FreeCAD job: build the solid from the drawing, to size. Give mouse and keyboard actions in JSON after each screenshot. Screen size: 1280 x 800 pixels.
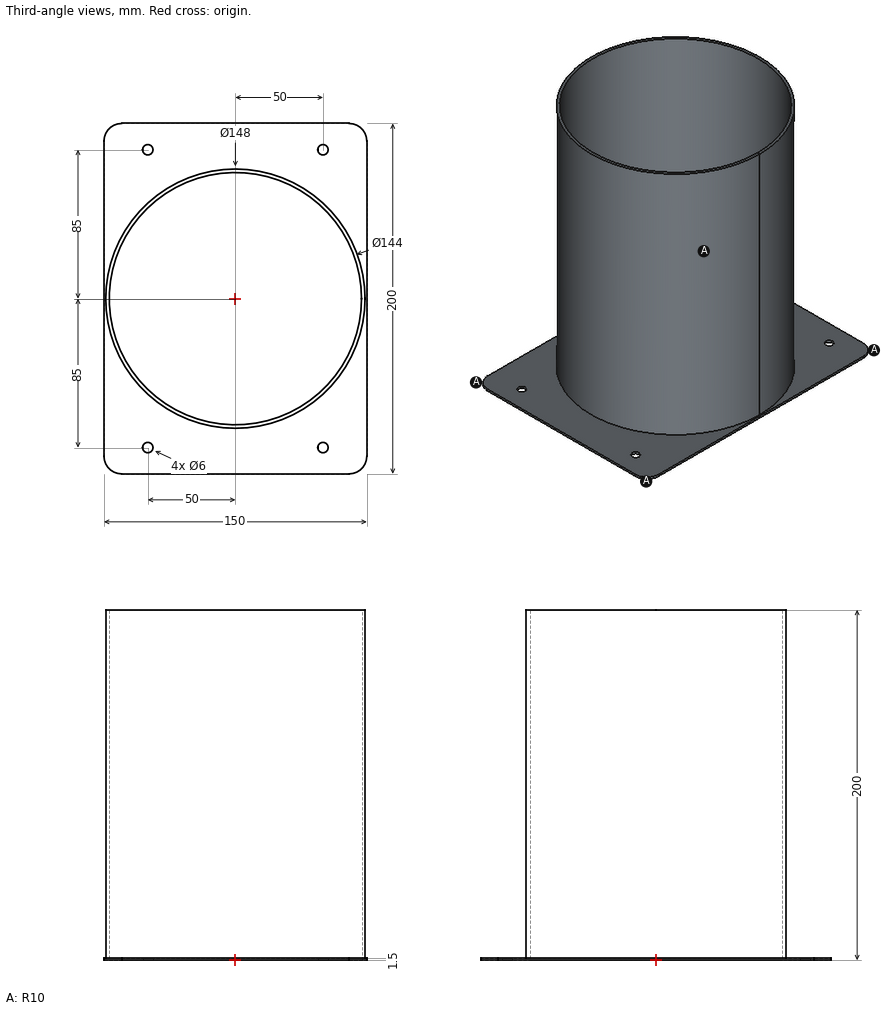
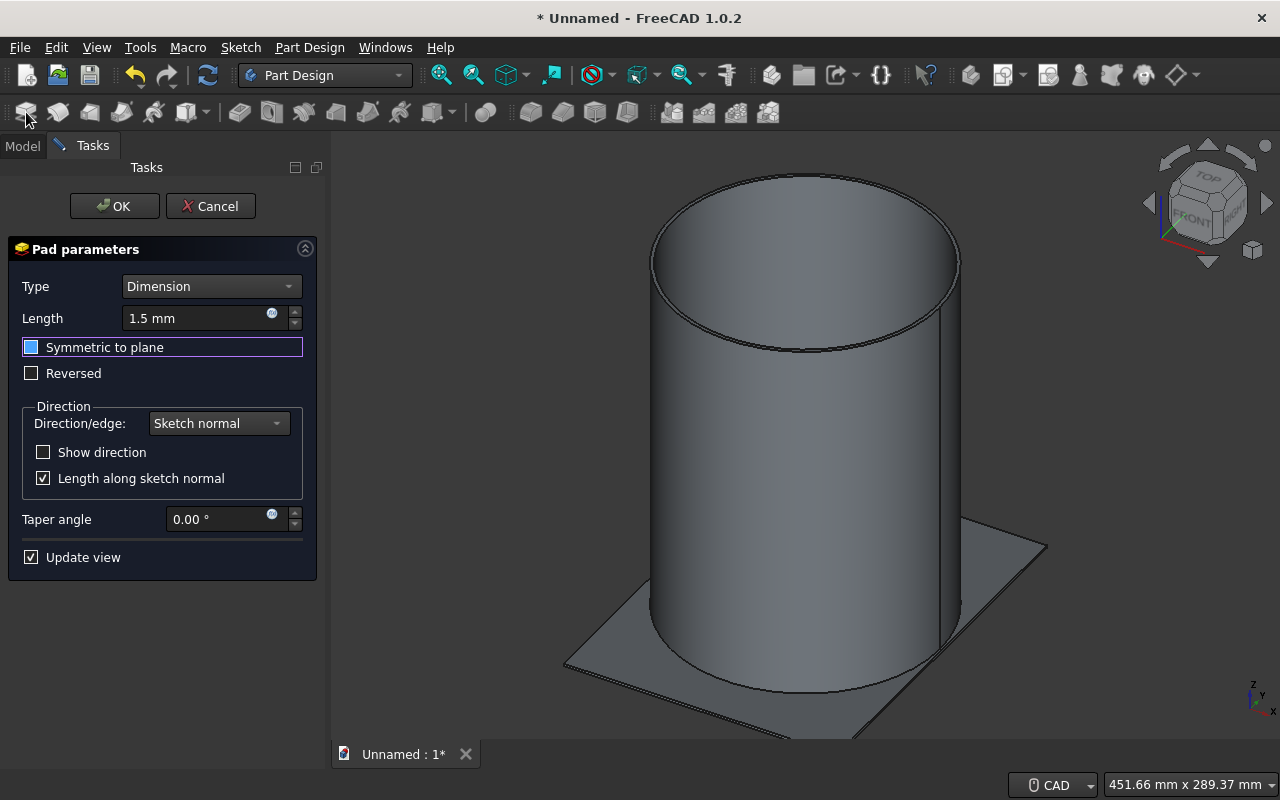
{"action": "left_click", "coordinate": [115, 206]}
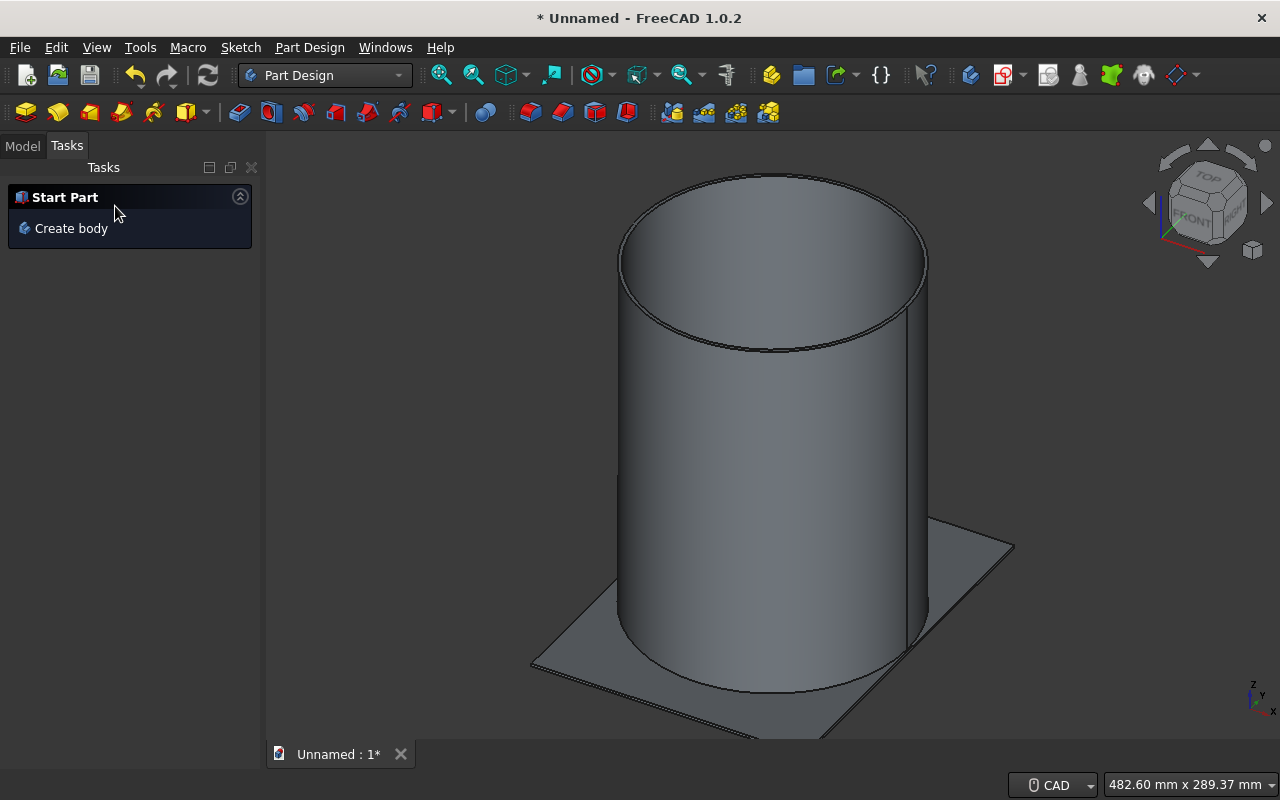
{"action": "left_click", "coordinate": [442, 76]}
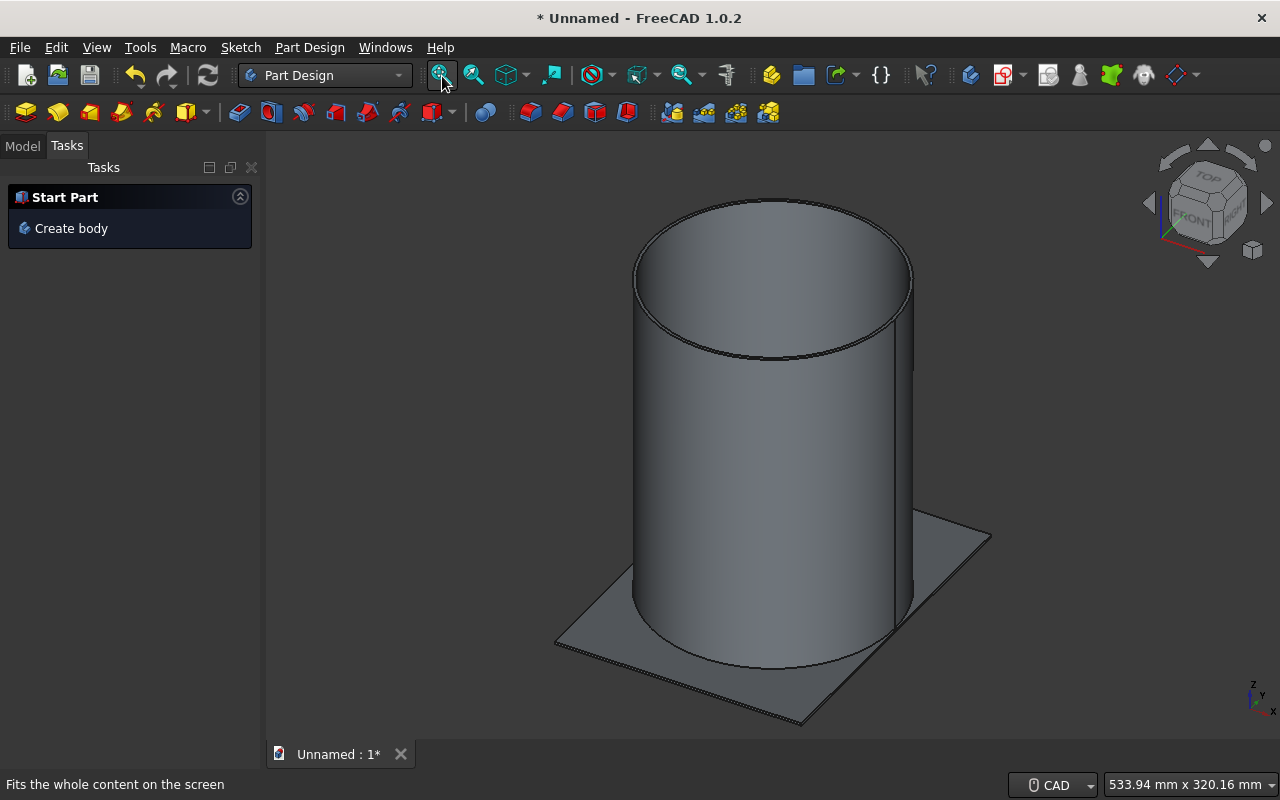
{"action": "scroll", "coordinate": [745, 453], "scroll_direction": "up", "scroll_amount": 14}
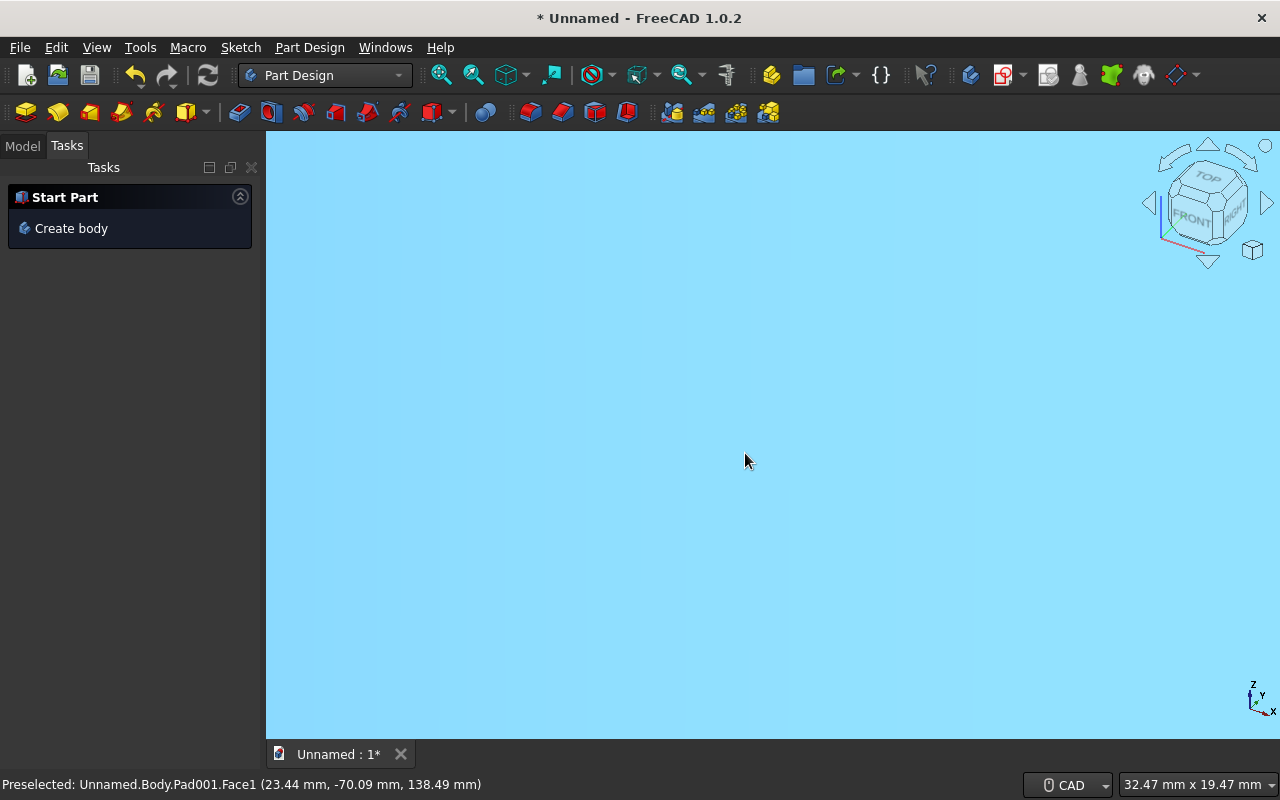
{"action": "left_click", "coordinate": [442, 76]}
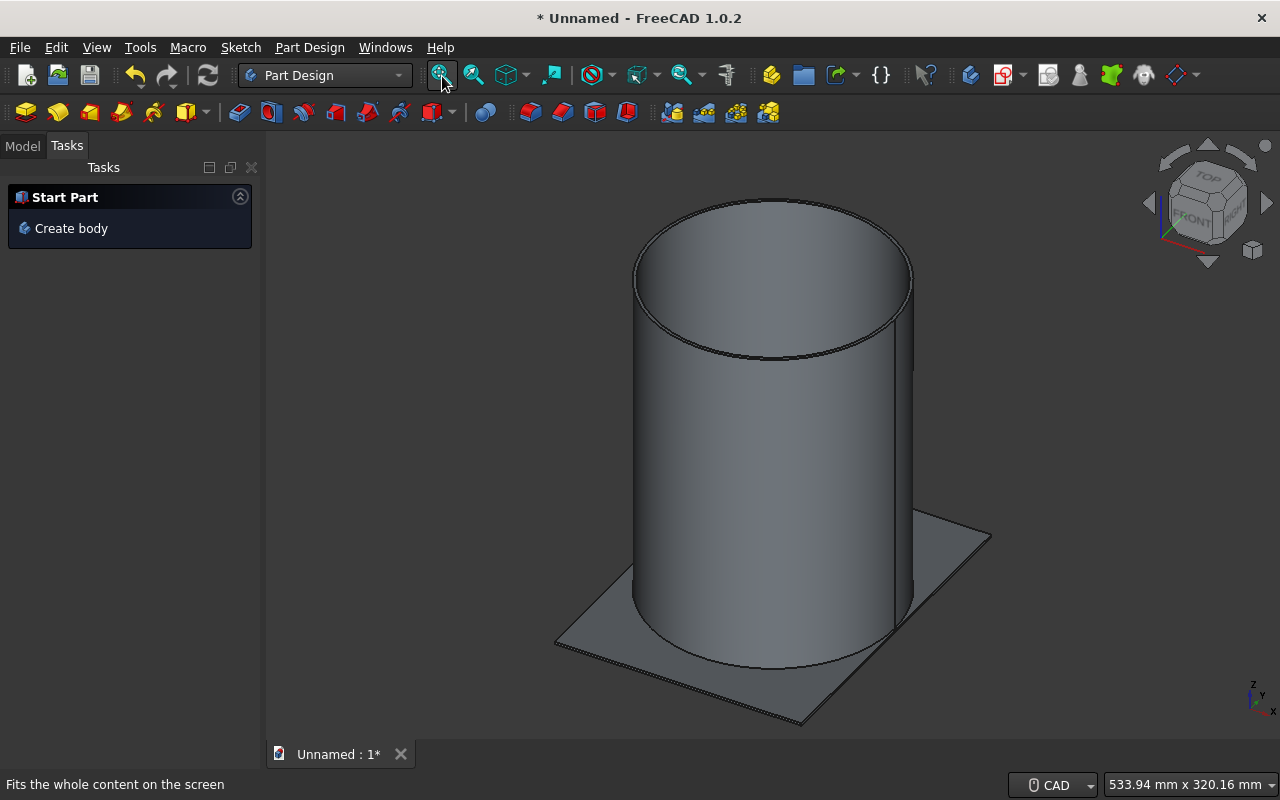
{"action": "key", "text": "0"}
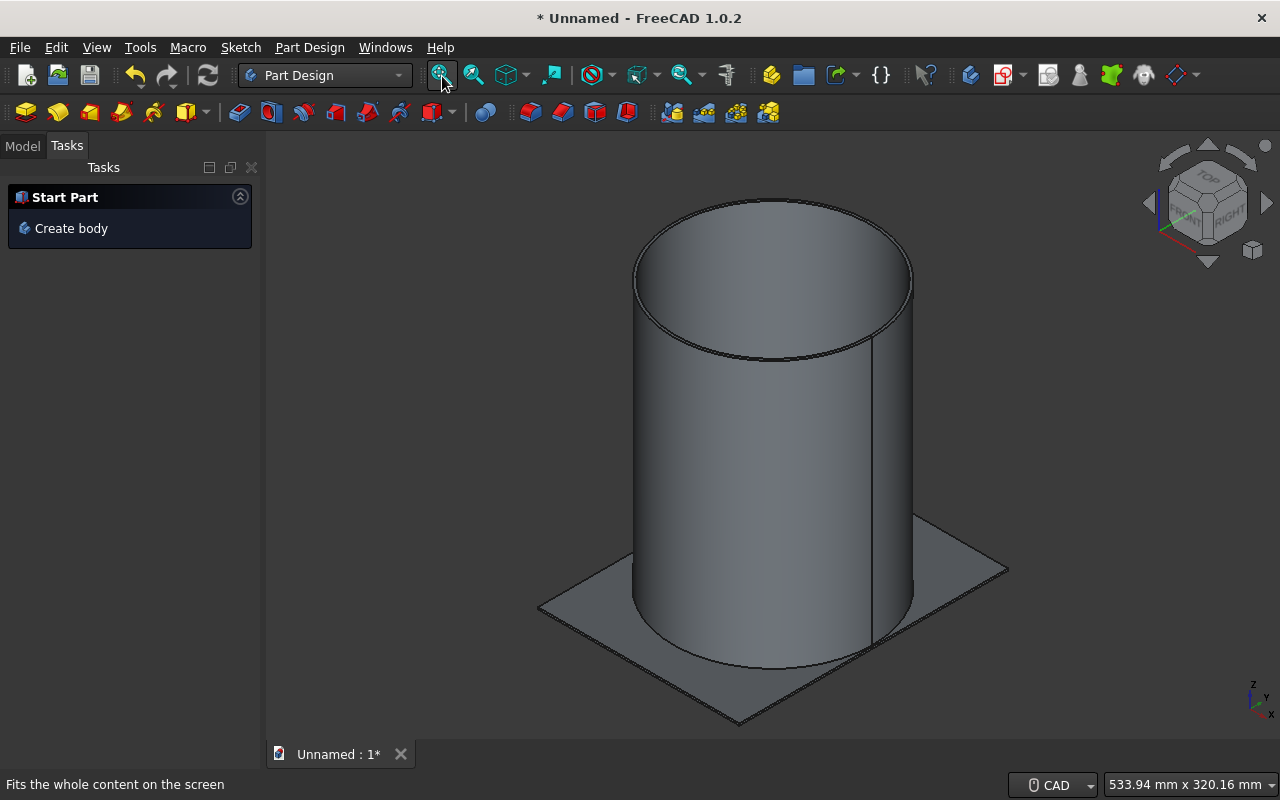
{"action": "scroll", "coordinate": [807, 452], "scroll_direction": "up", "scroll_amount": 14}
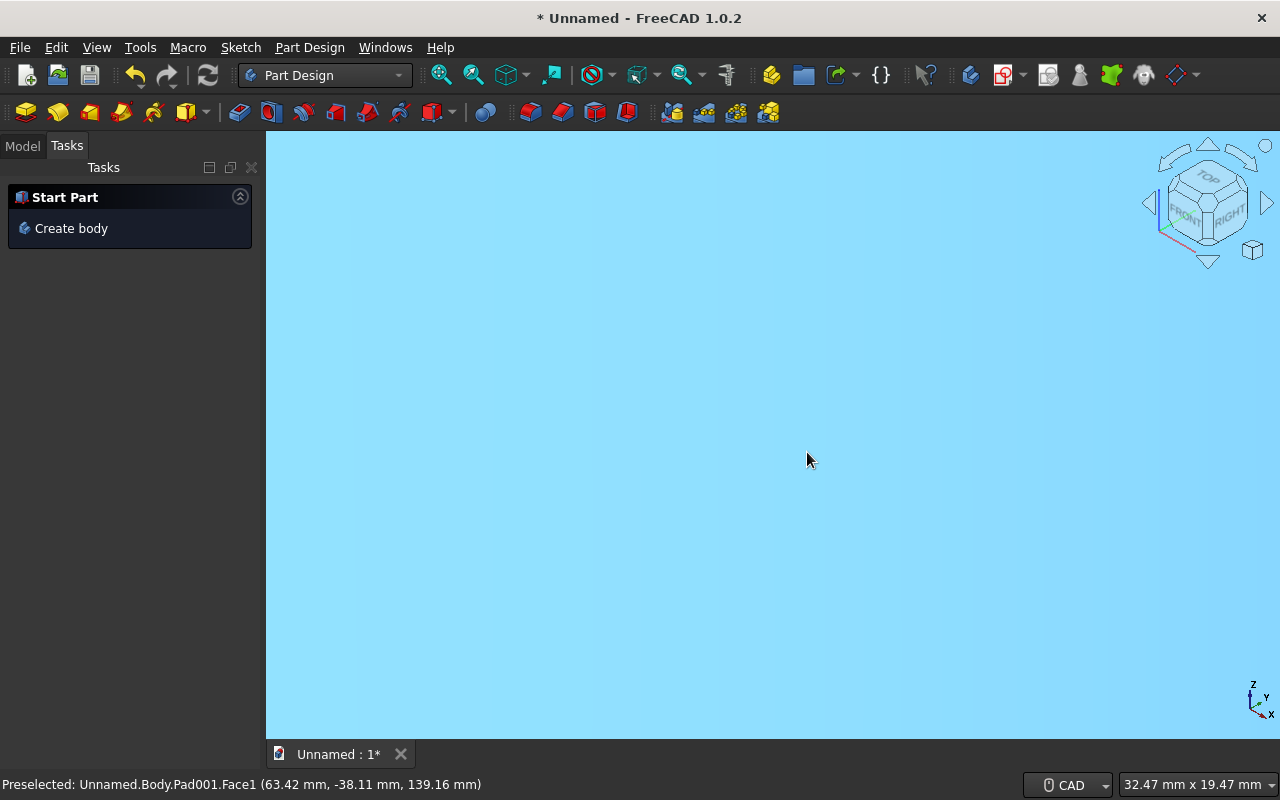
{"action": "left_click", "coordinate": [442, 76]}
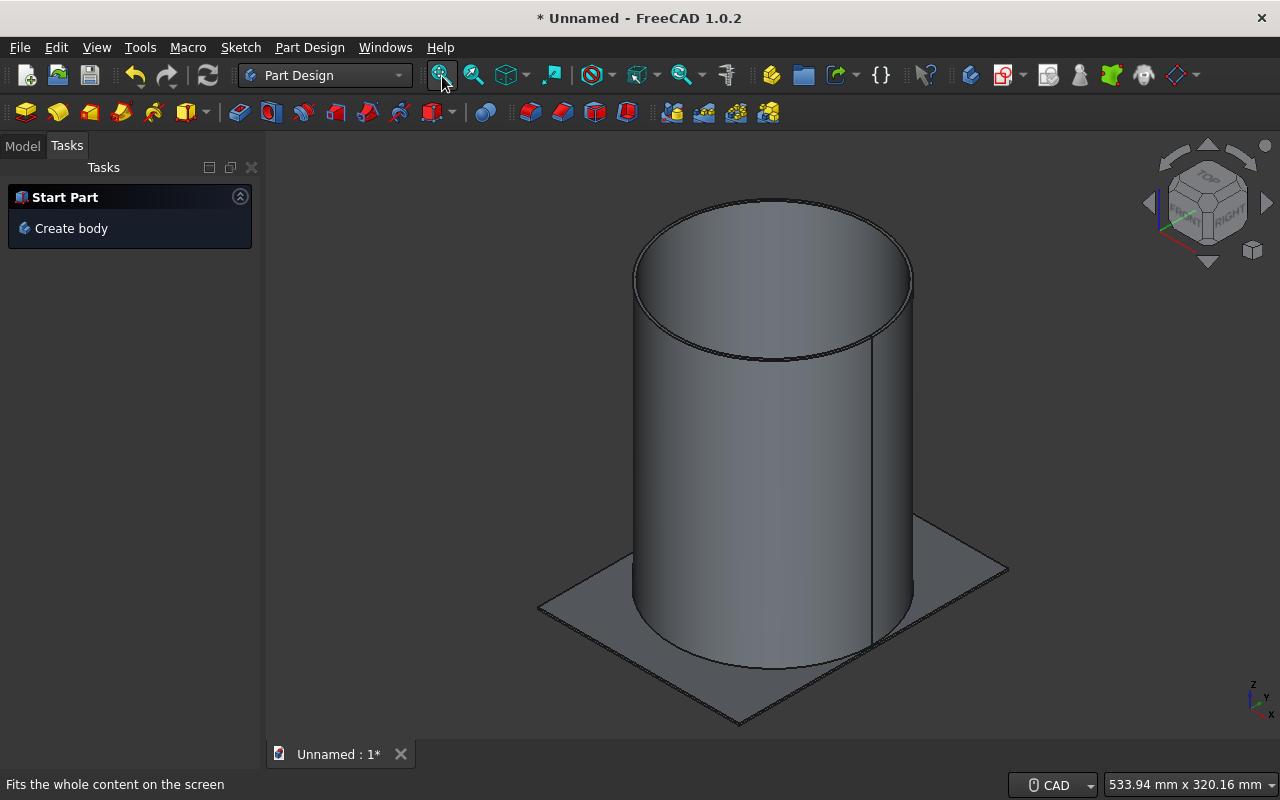
{"action": "key", "text": "2"}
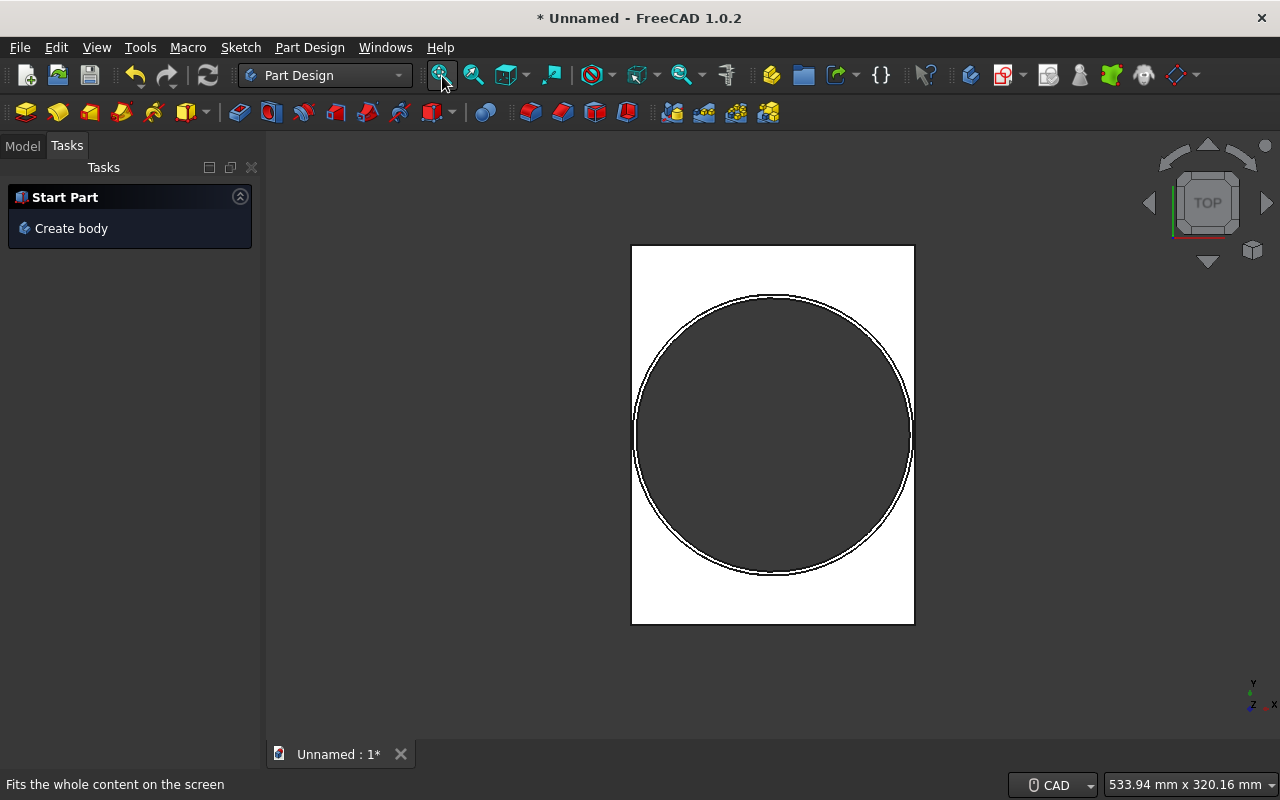
{"action": "scroll", "coordinate": [631, 244], "scroll_direction": "up", "scroll_amount": 14}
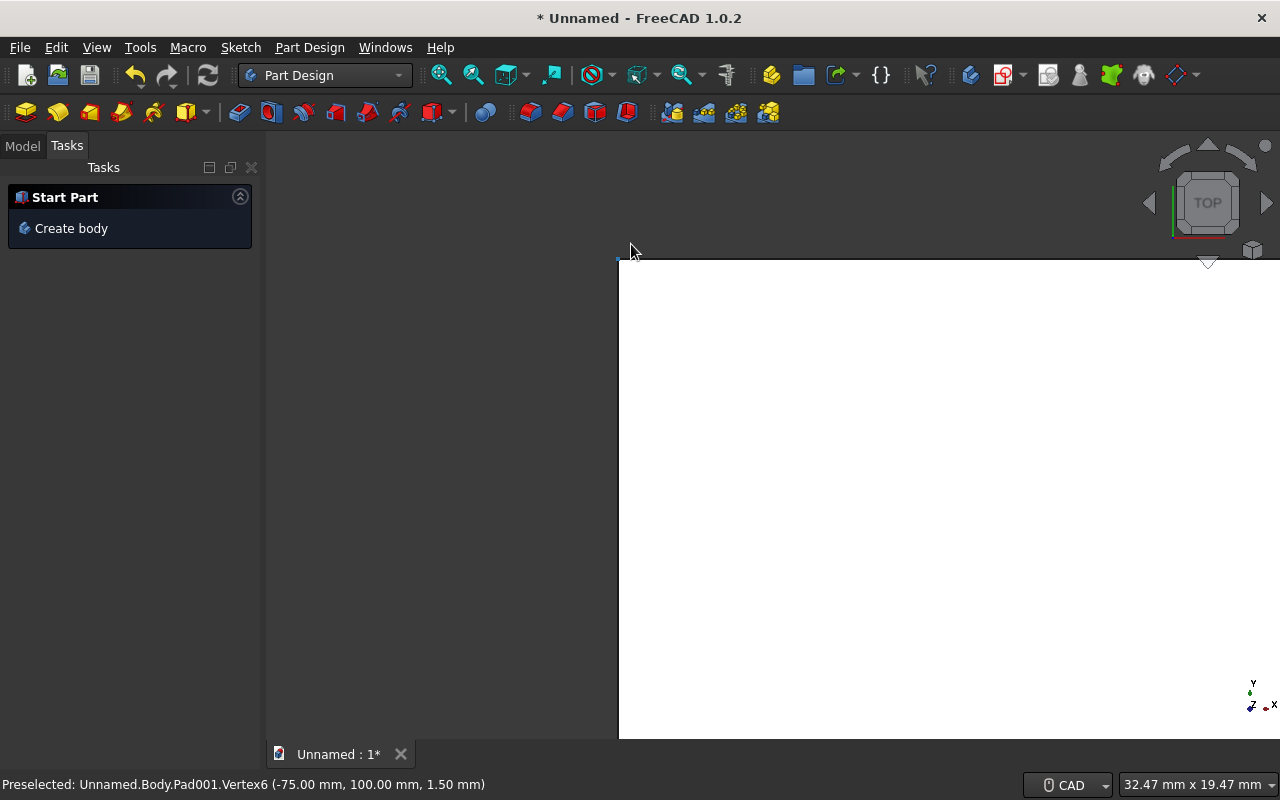
{"action": "left_click", "coordinate": [442, 76]}